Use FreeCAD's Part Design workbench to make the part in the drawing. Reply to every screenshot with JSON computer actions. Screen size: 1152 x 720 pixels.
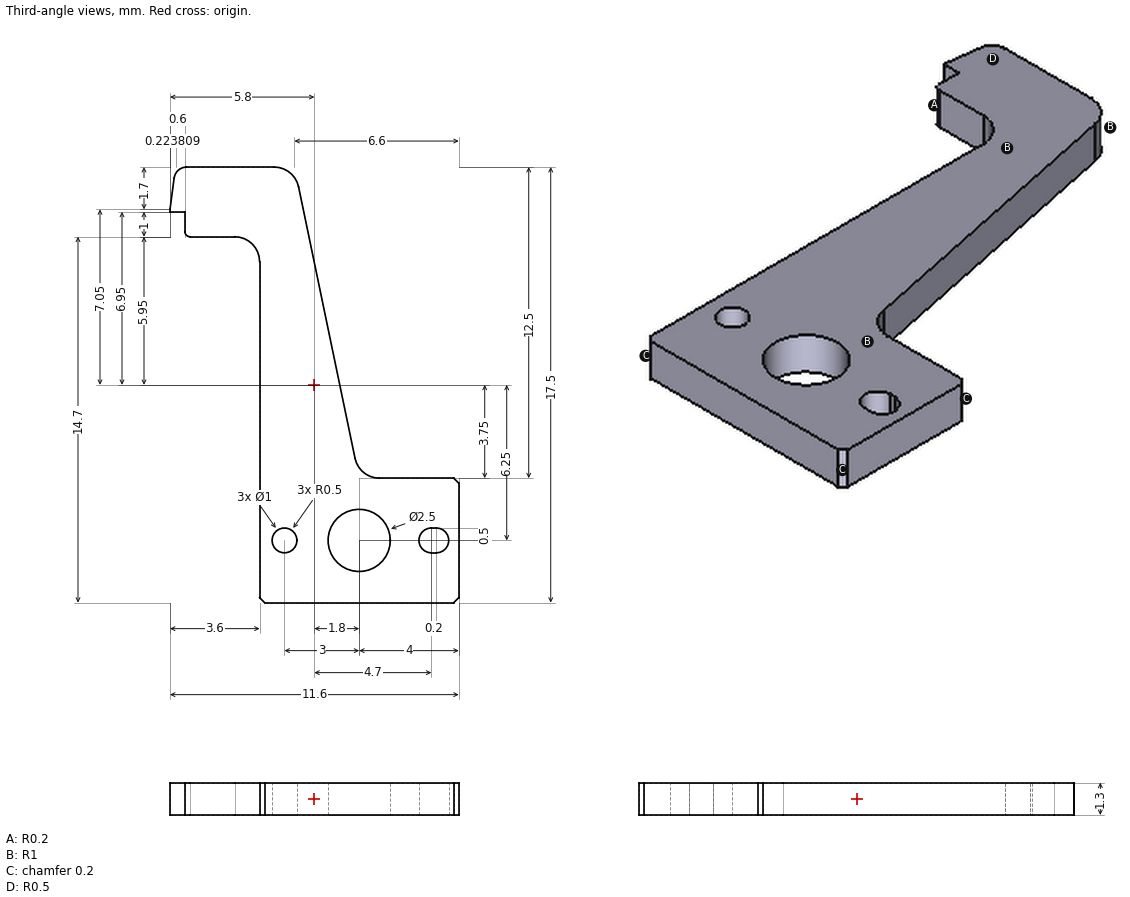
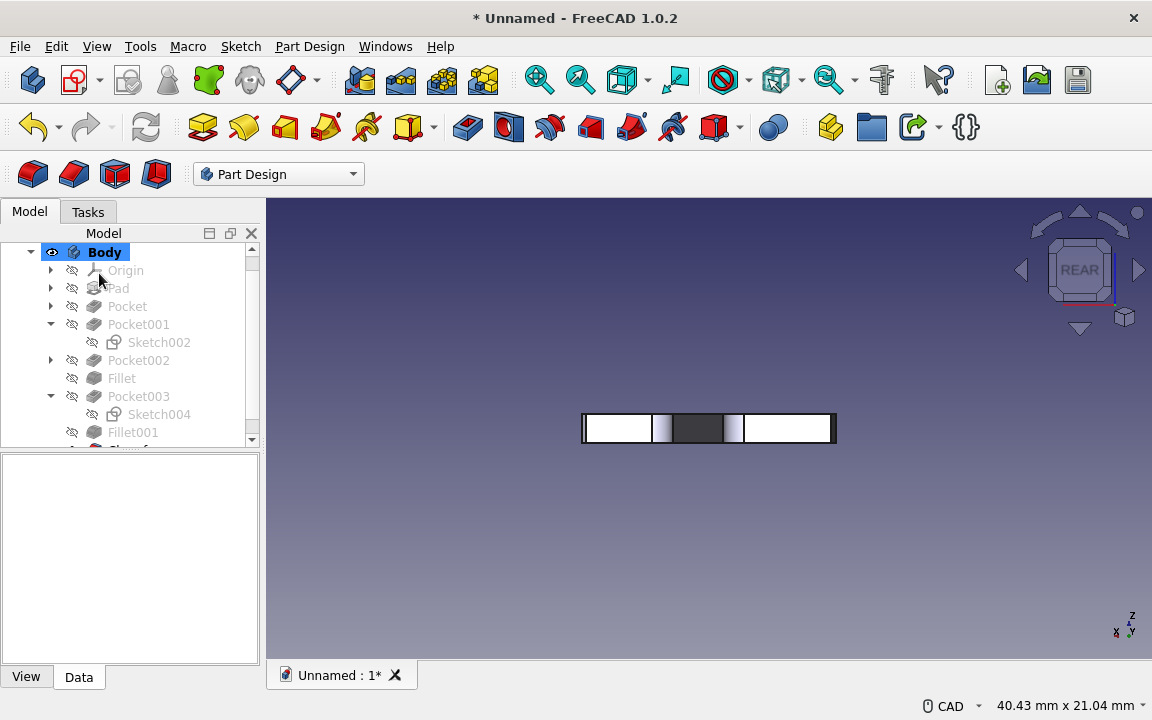
{"action": "key", "text": "v f"}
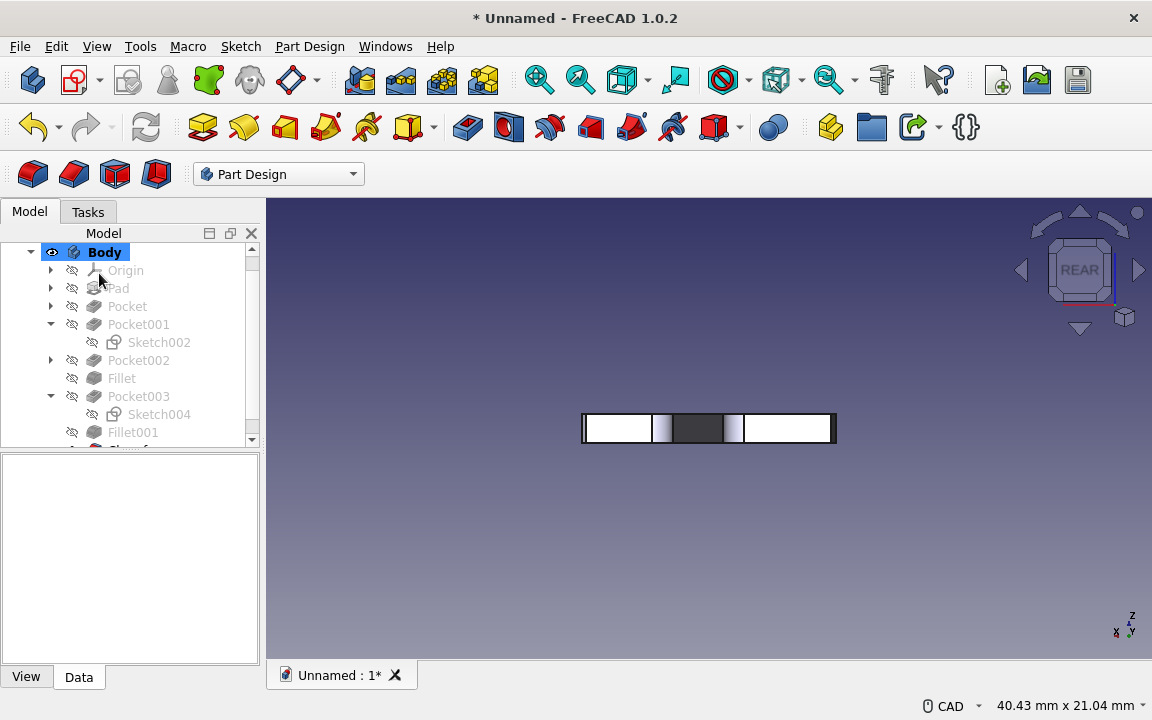
{"action": "left_click", "coordinate": [831, 428]}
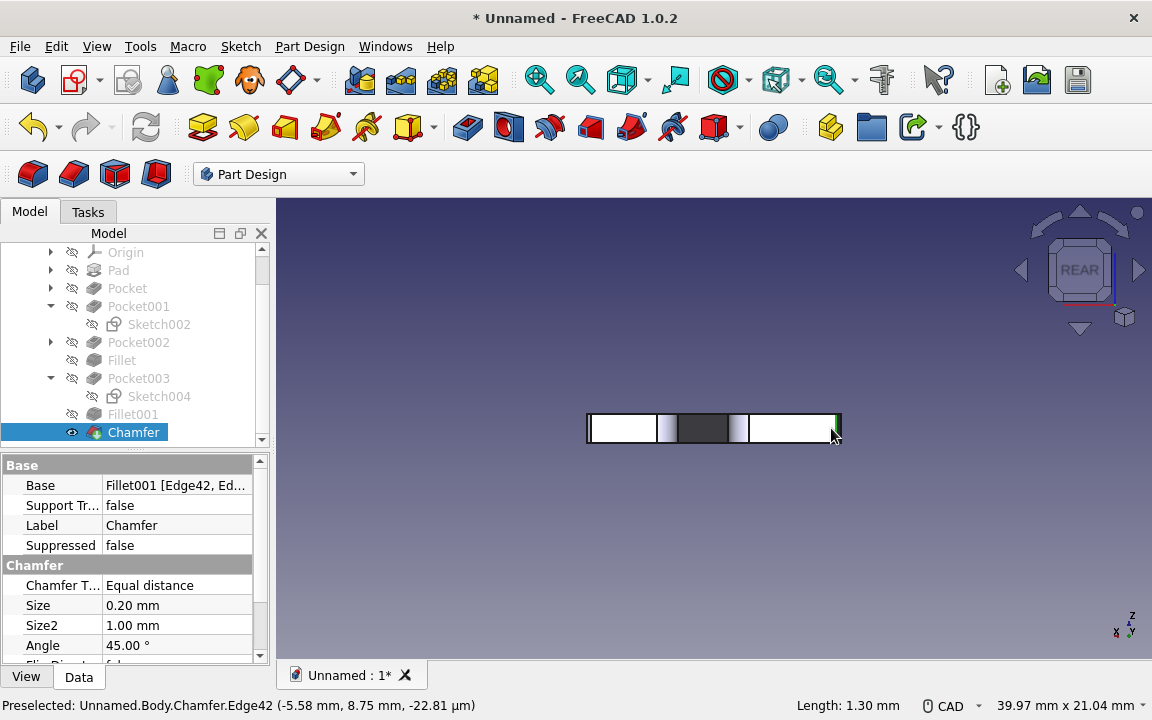
{"action": "left_click", "coordinate": [33, 174]}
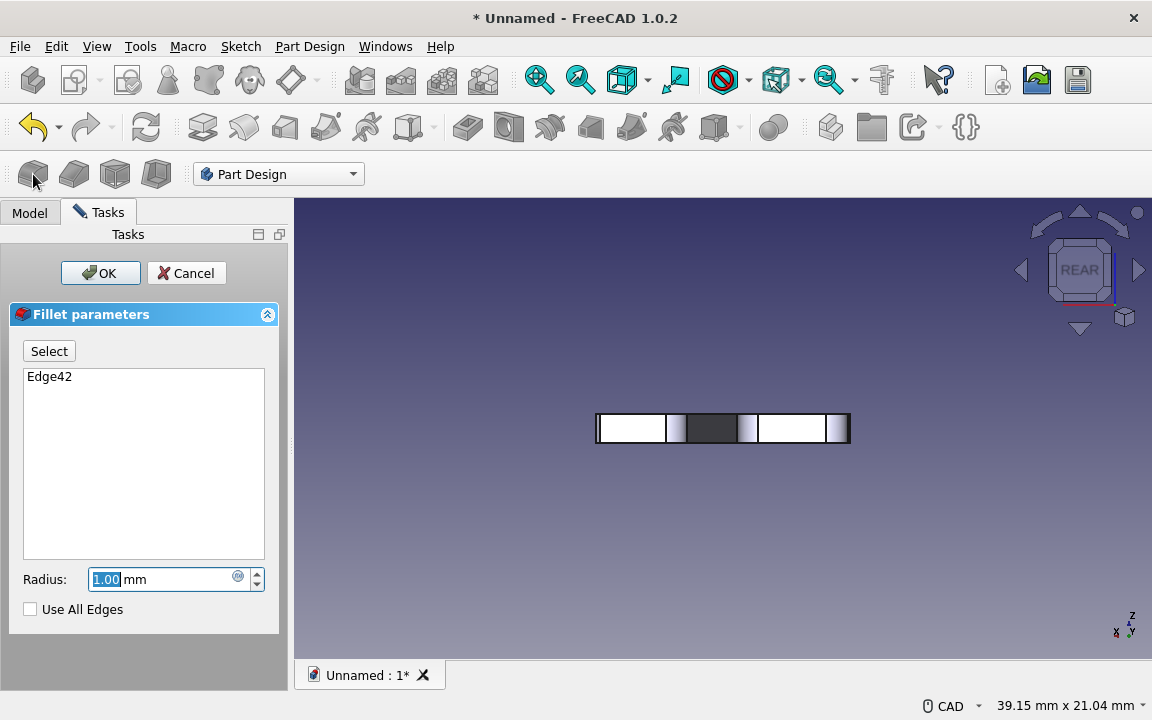
{"action": "type", "text": "0.5"}
{"action": "key", "text": "Tab"}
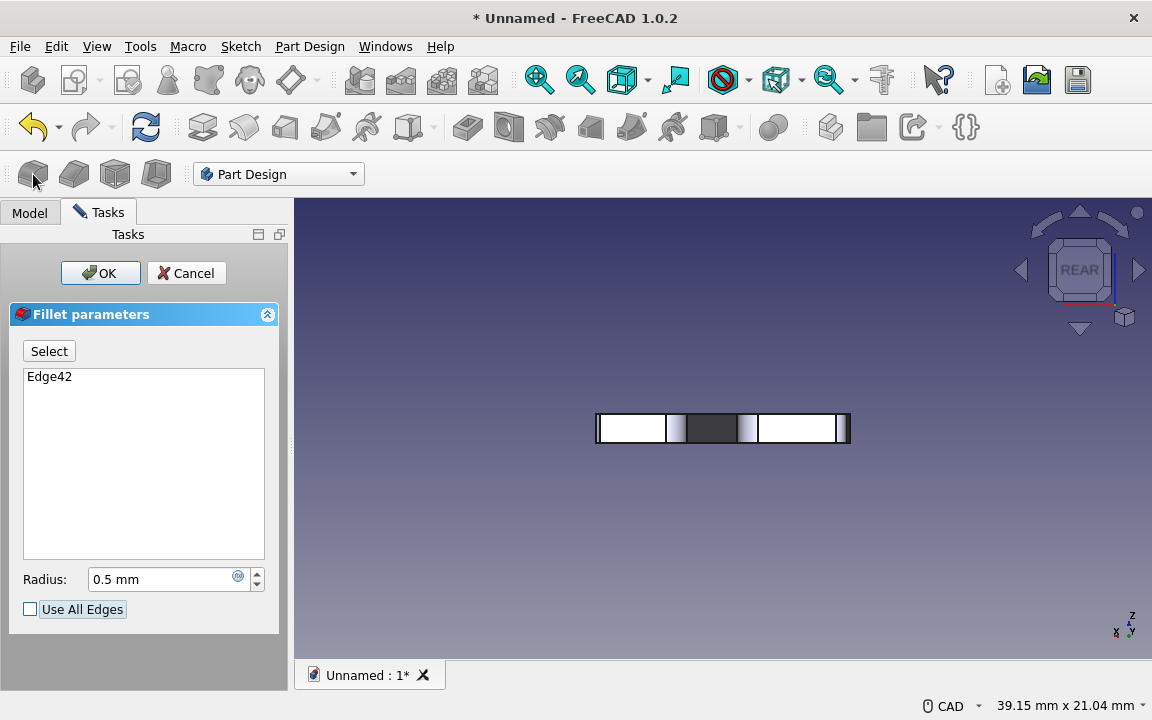
{"action": "left_click", "coordinate": [101, 273]}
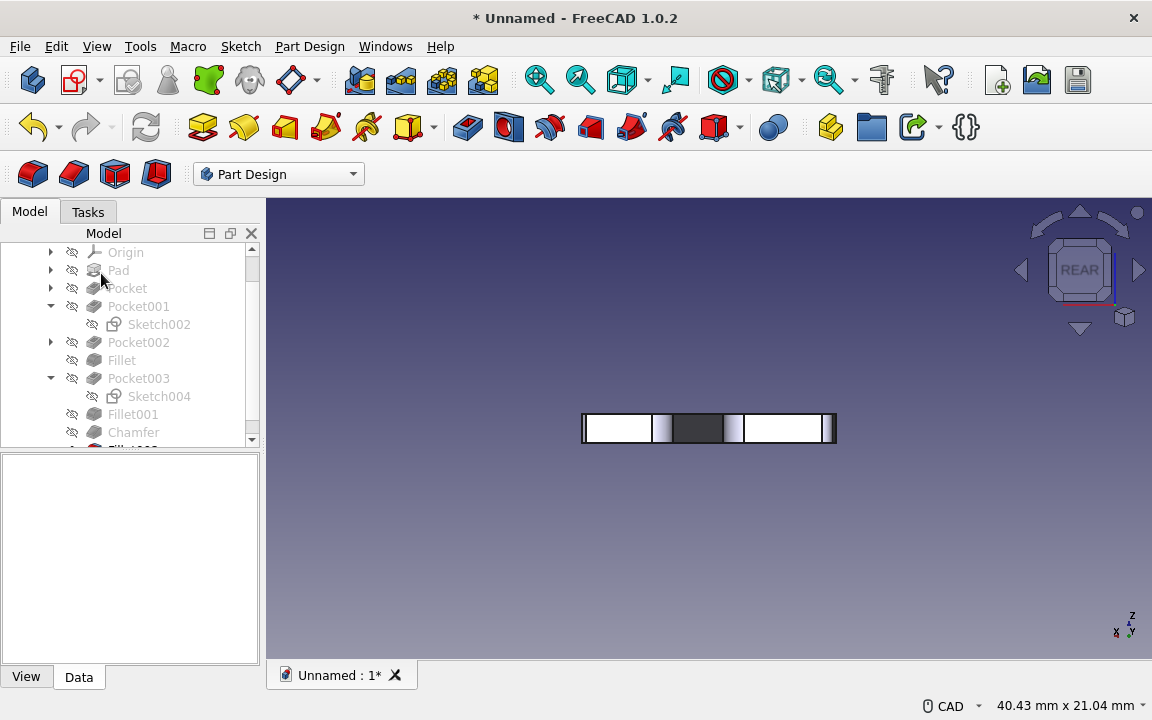
{"action": "key", "text": "0"}